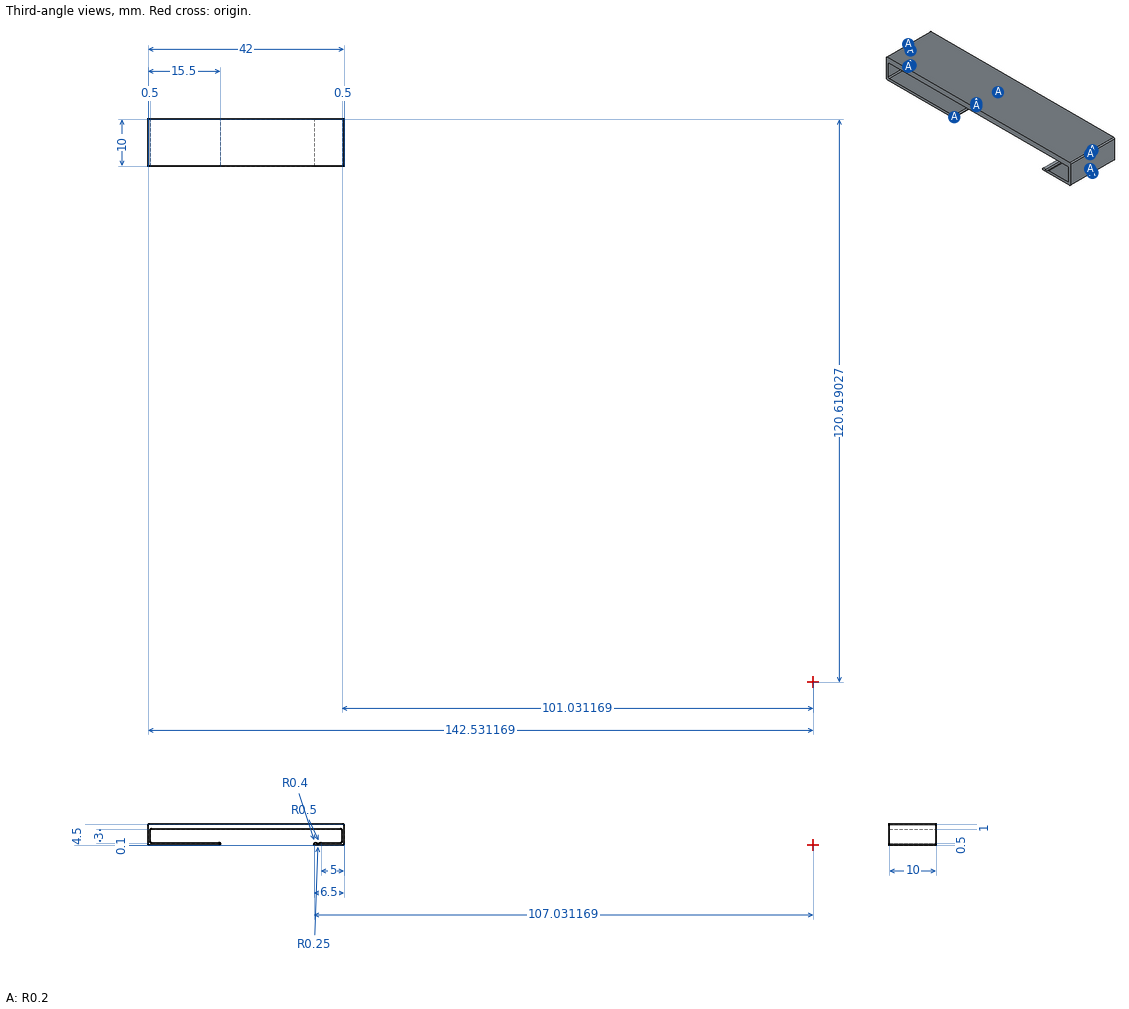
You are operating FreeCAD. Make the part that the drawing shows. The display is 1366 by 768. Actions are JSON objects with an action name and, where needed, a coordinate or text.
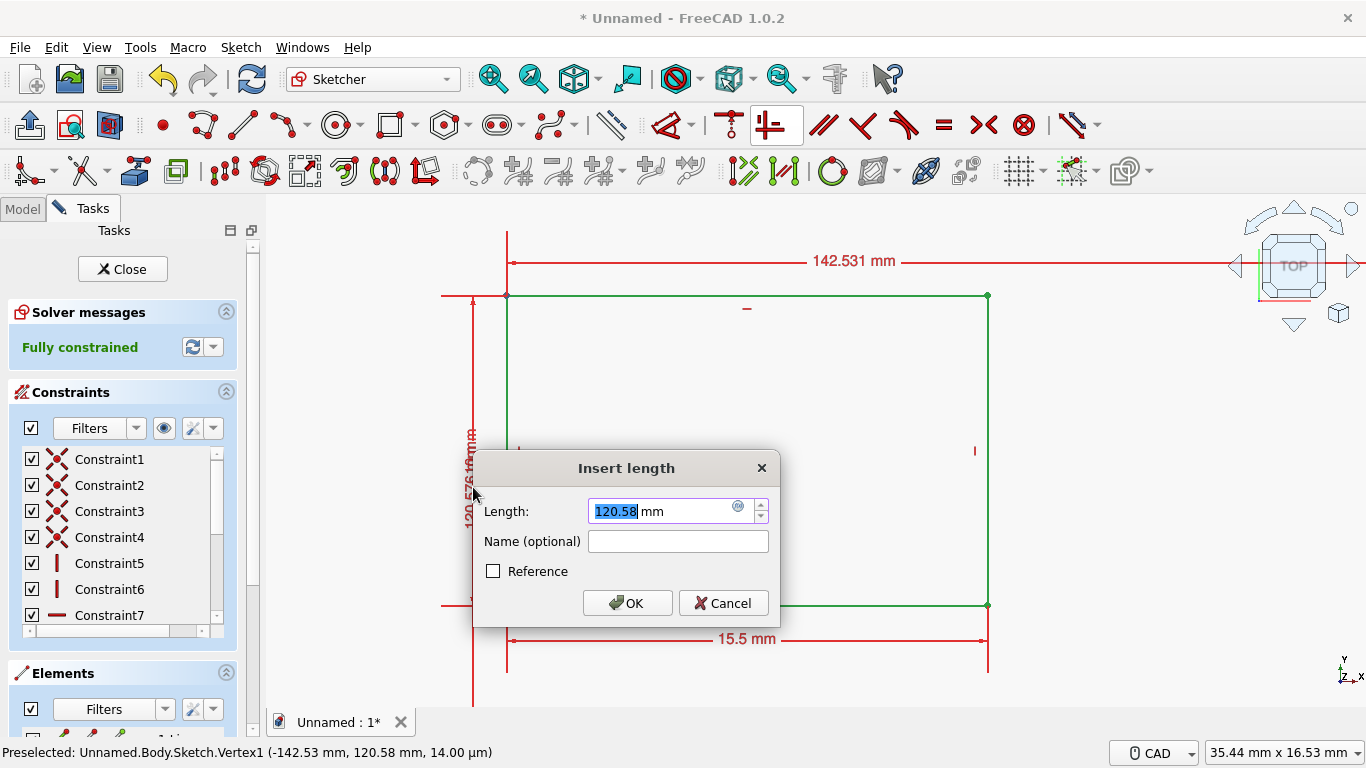
{"action": "type", "text": "120.619027"}
{"action": "key", "text": "Return"}
{"action": "key", "text": "Escape"}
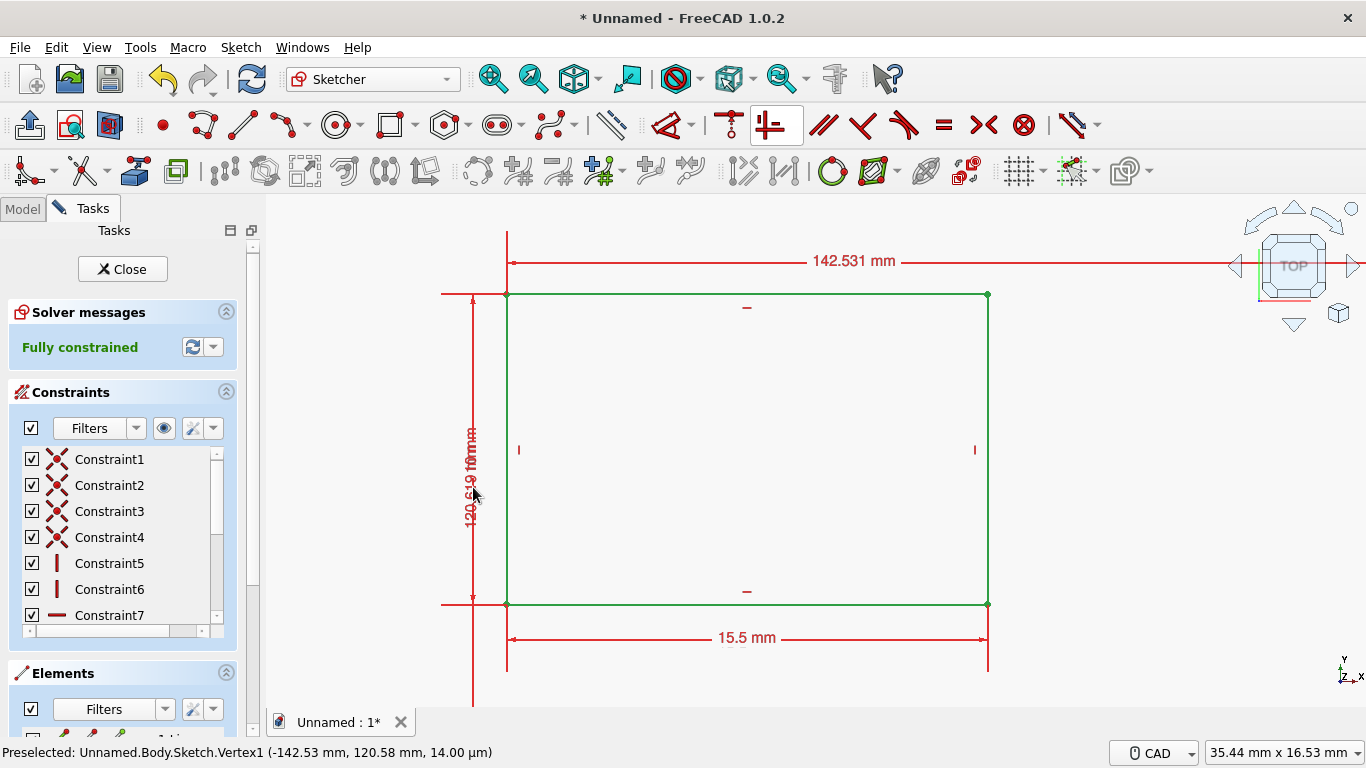
{"action": "left_click", "coordinate": [123, 269]}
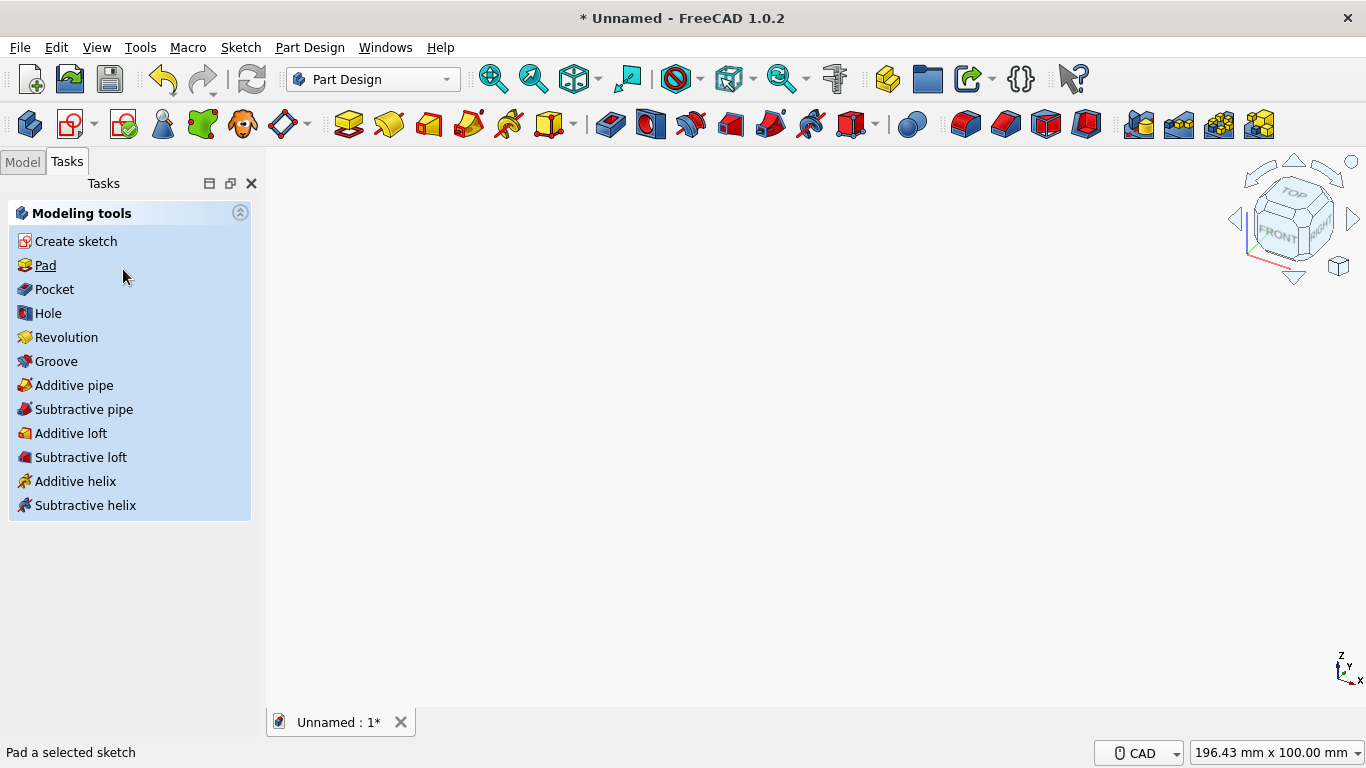
{"action": "left_click", "coordinate": [350, 124]}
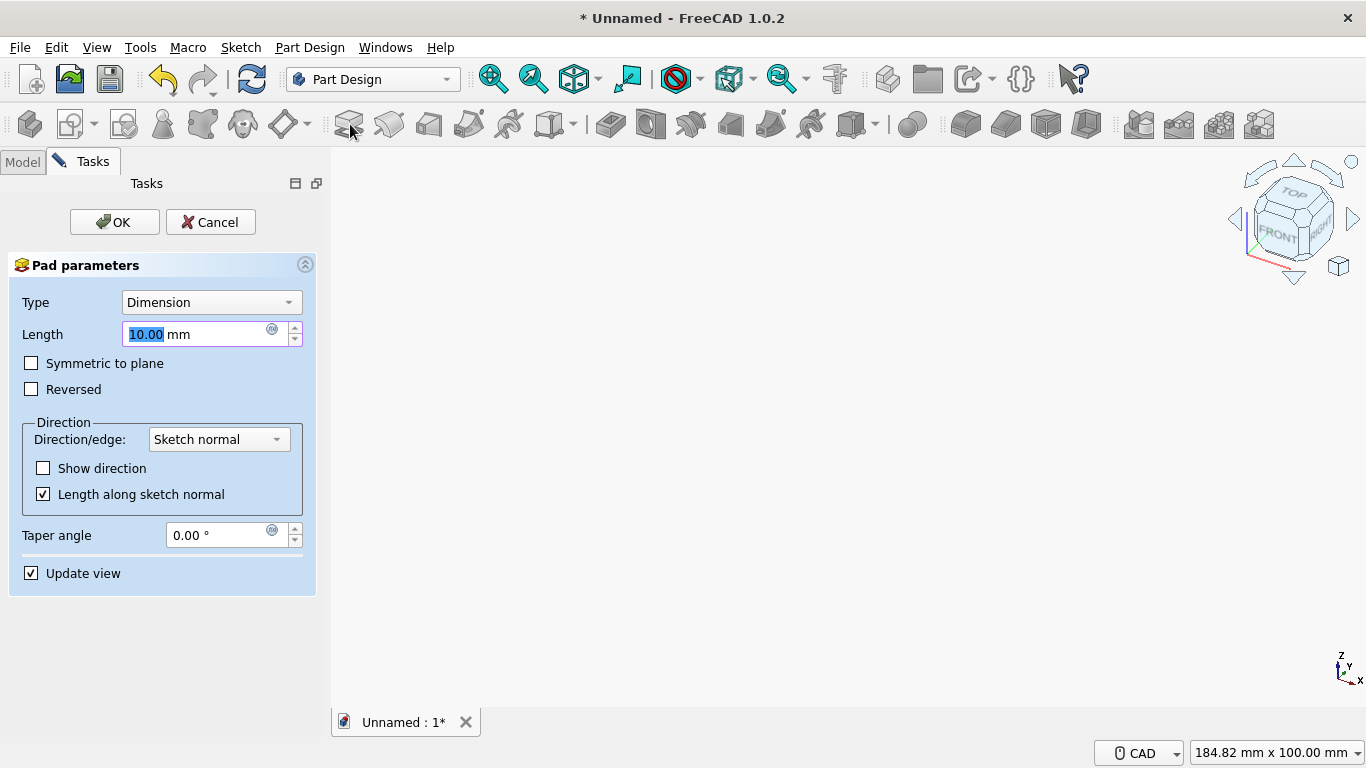
{"action": "type", "text": "0.5"}
{"action": "key", "text": "Tab"}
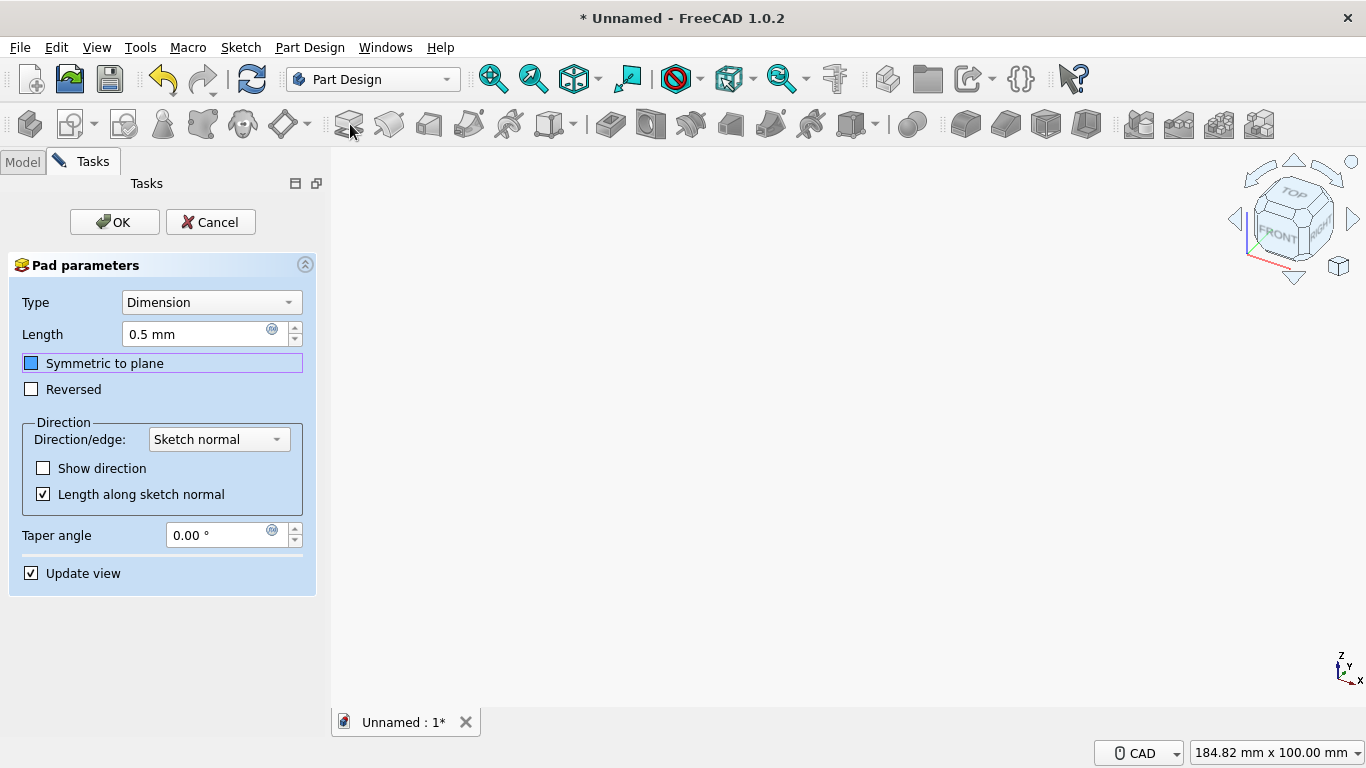
{"action": "left_click", "coordinate": [115, 222]}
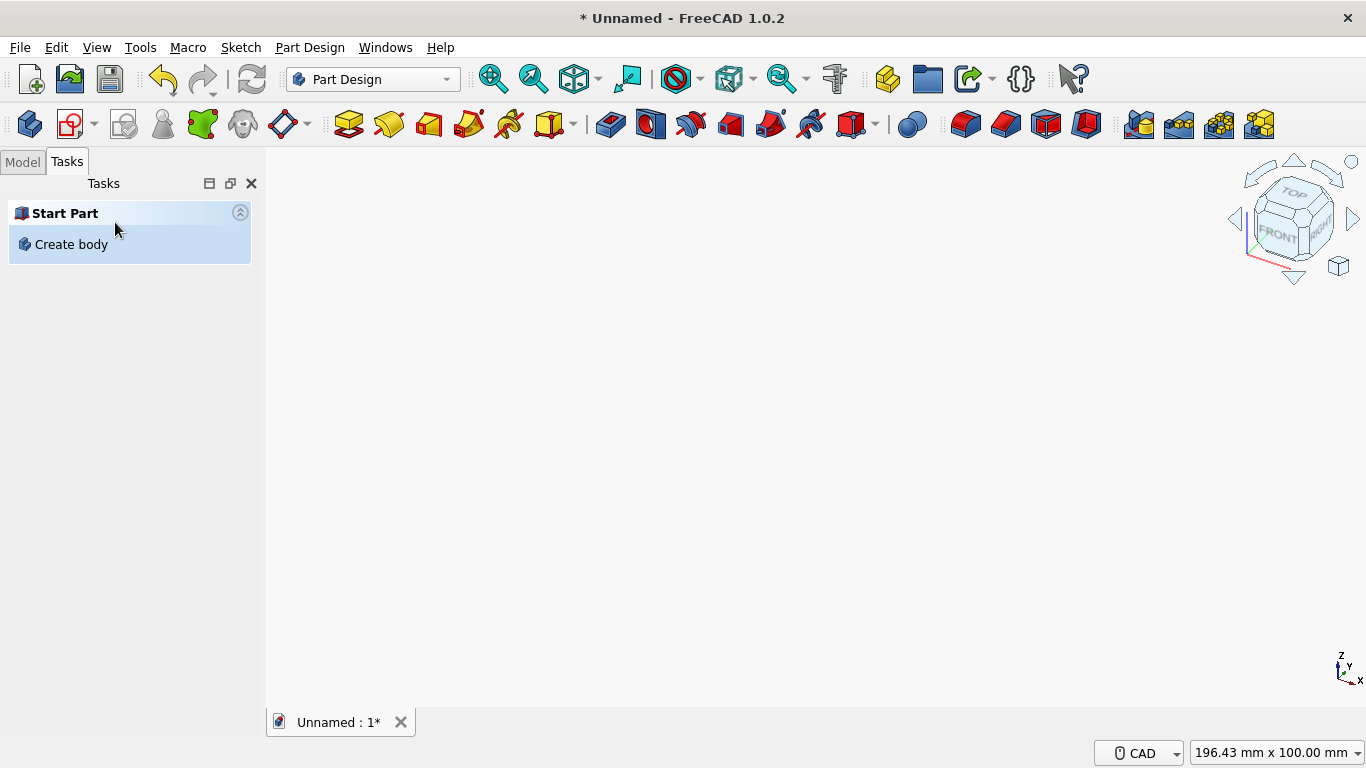
{"action": "left_click", "coordinate": [494, 80]}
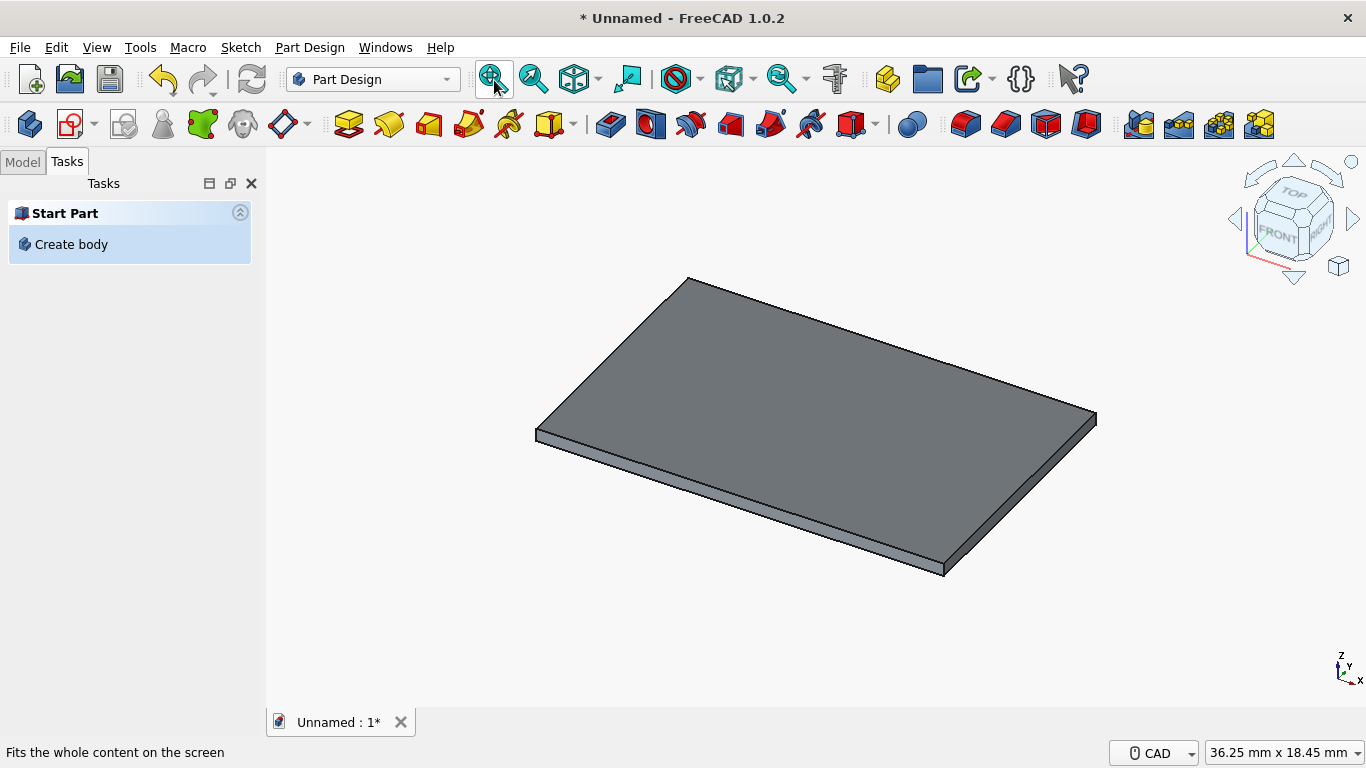
{"action": "left_click", "coordinate": [874, 439]}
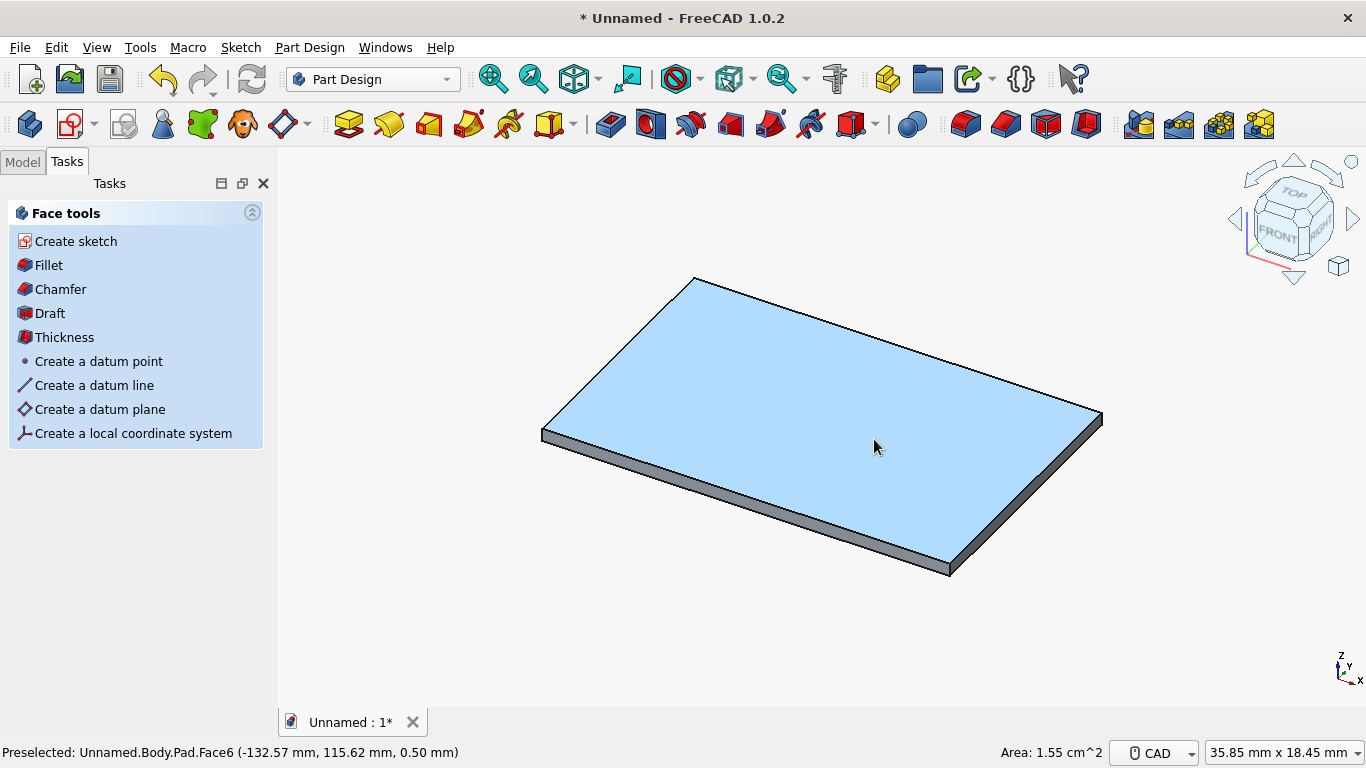
{"action": "left_click", "coordinate": [70, 124]}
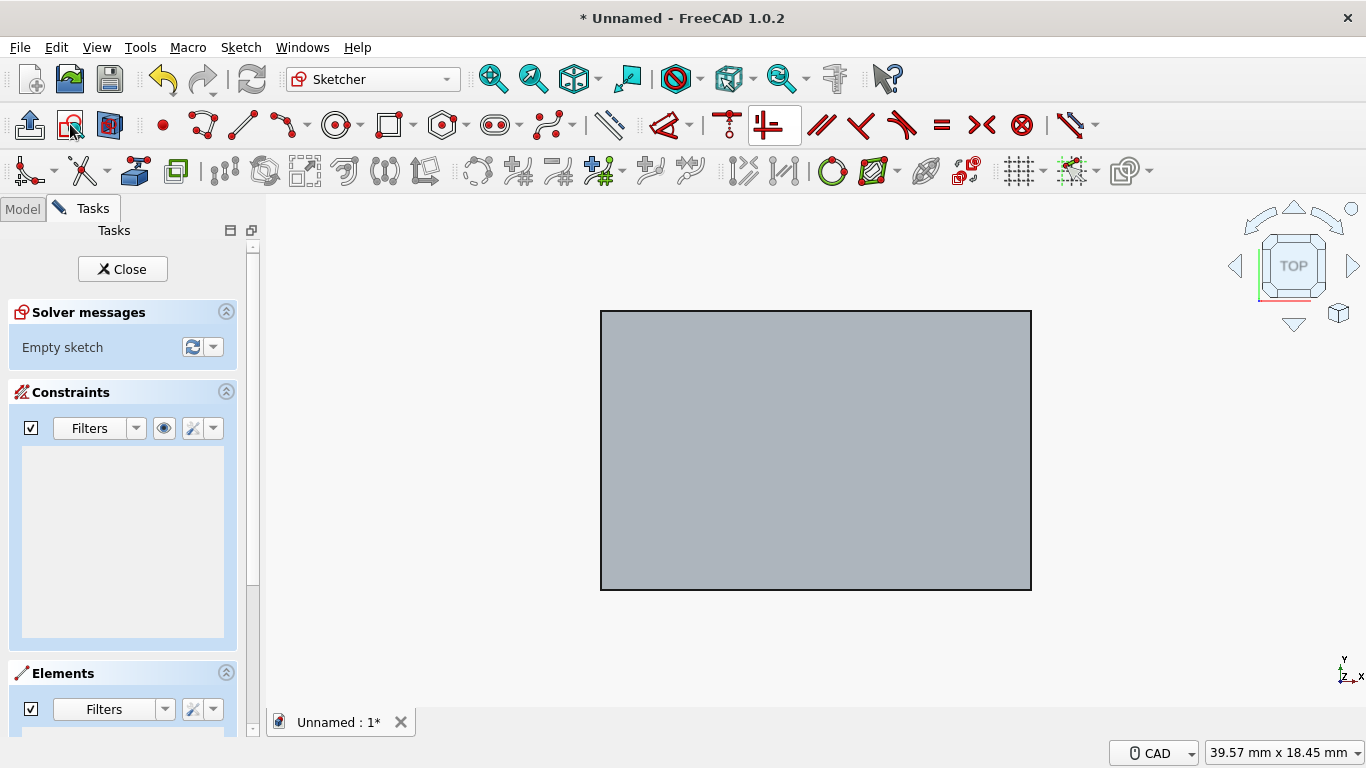
{"action": "left_click", "coordinate": [390, 126]}